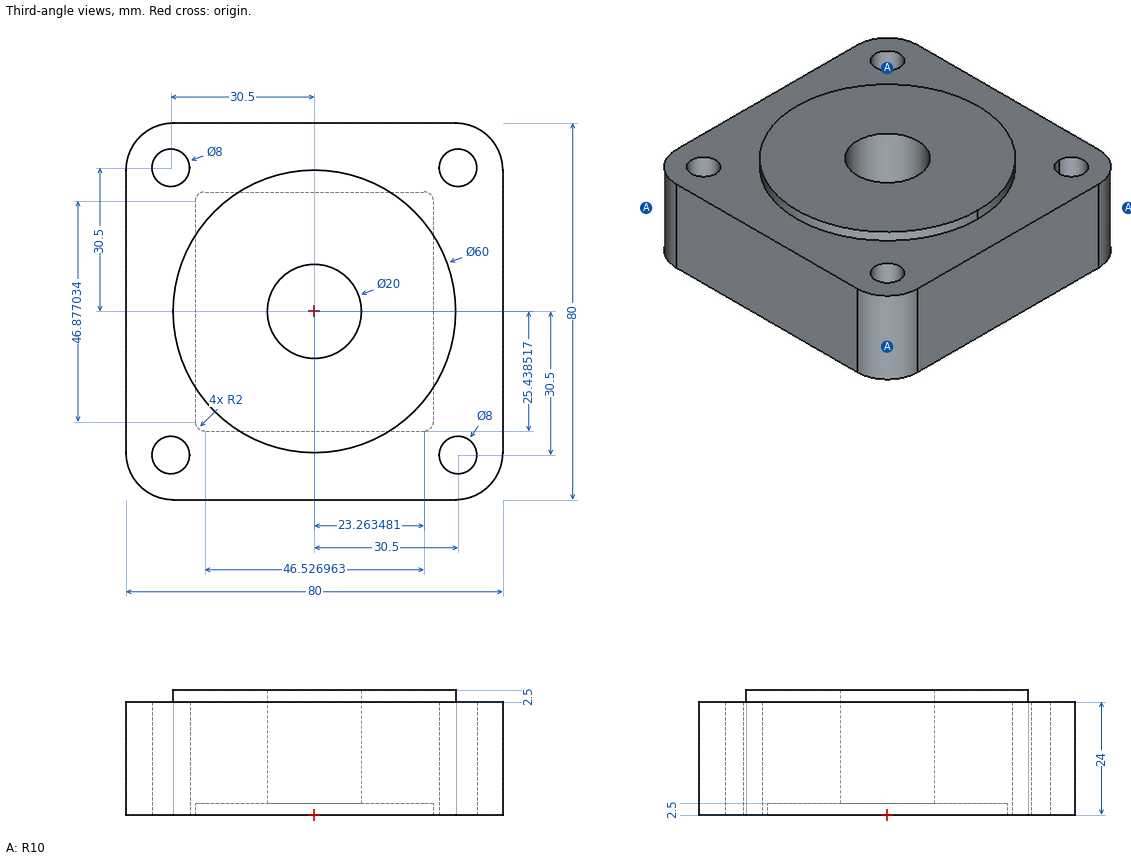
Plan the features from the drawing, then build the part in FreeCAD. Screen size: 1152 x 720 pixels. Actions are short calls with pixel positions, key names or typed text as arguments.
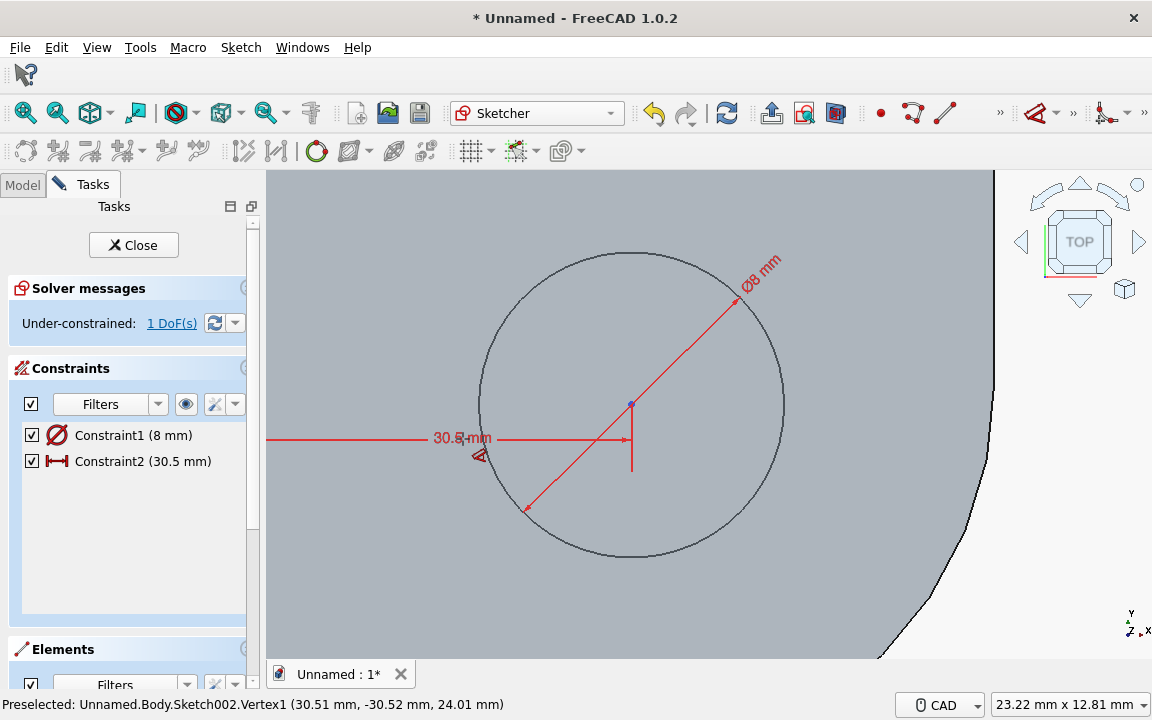
click(632, 405)
click(666, 301)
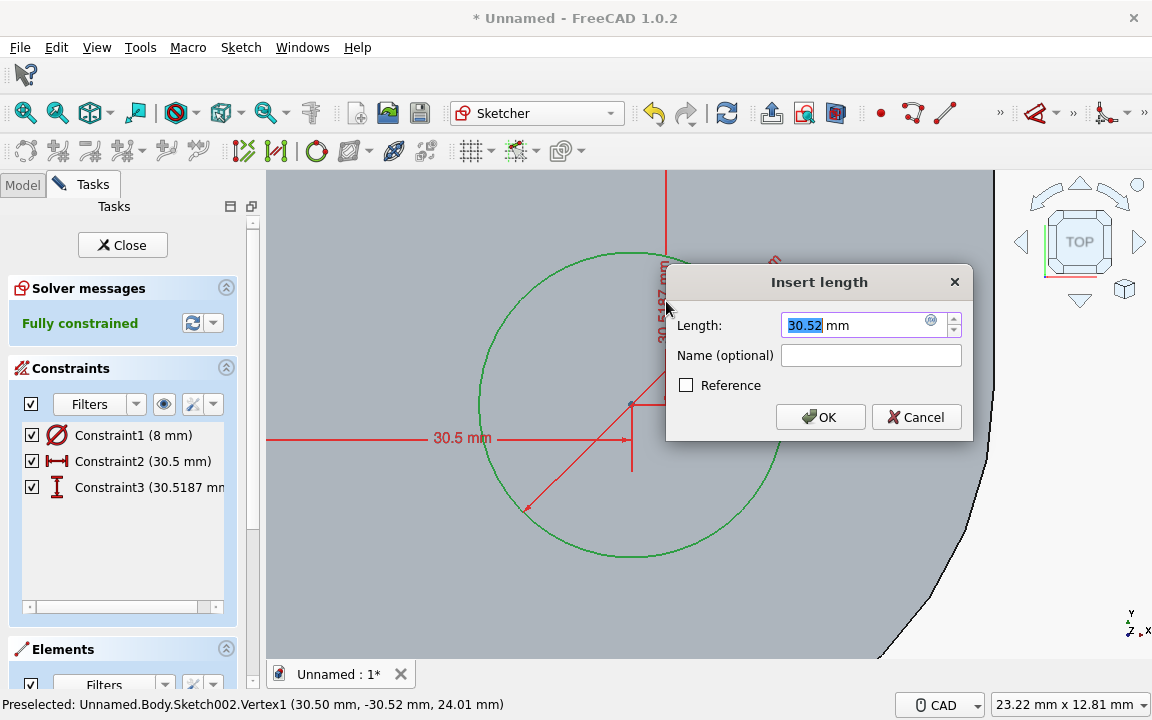
text(30.5)
key(Return)
key(Escape)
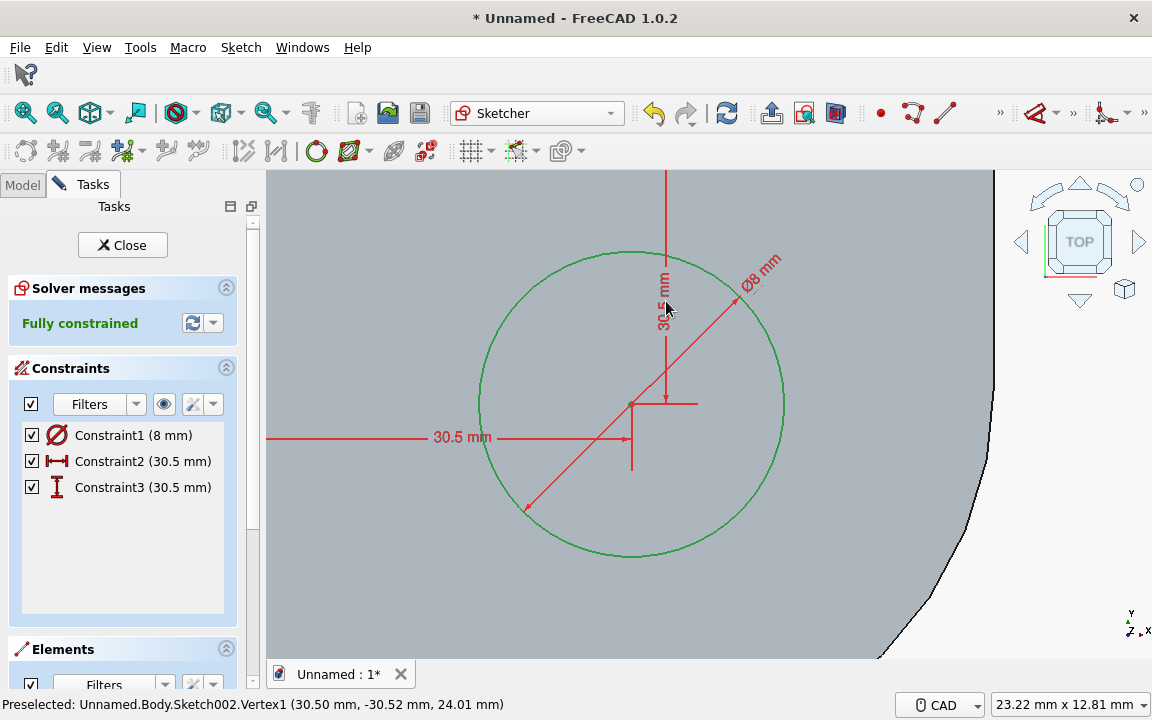
click(123, 245)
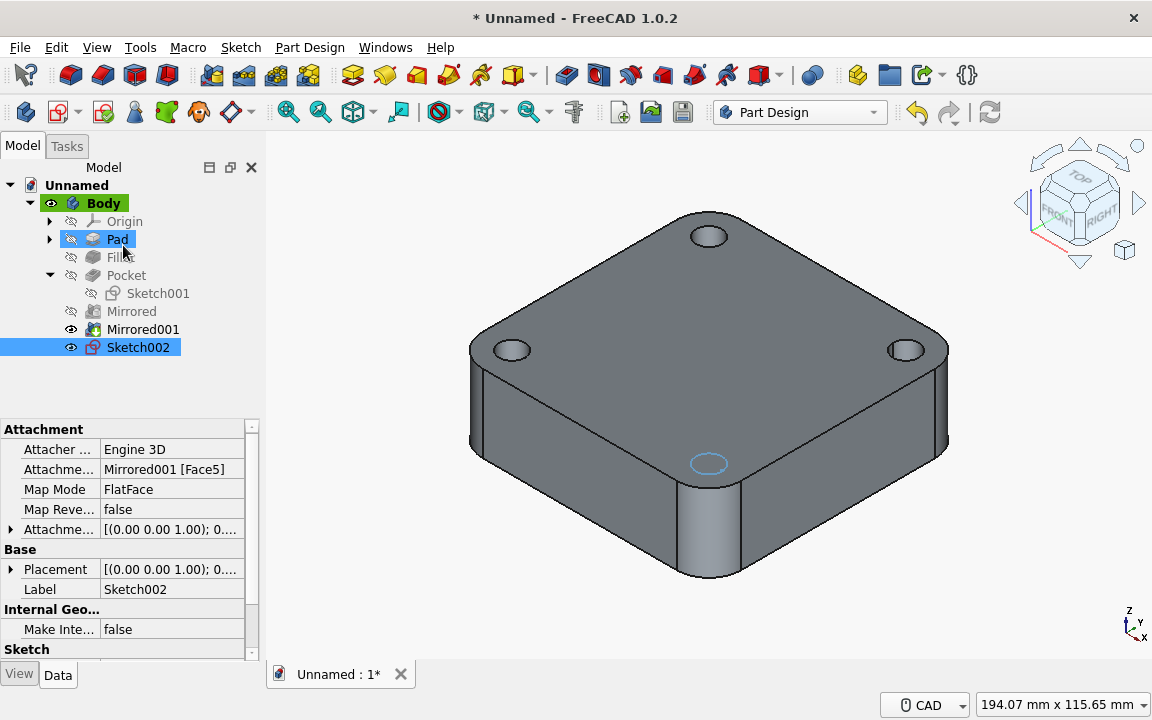
click(568, 76)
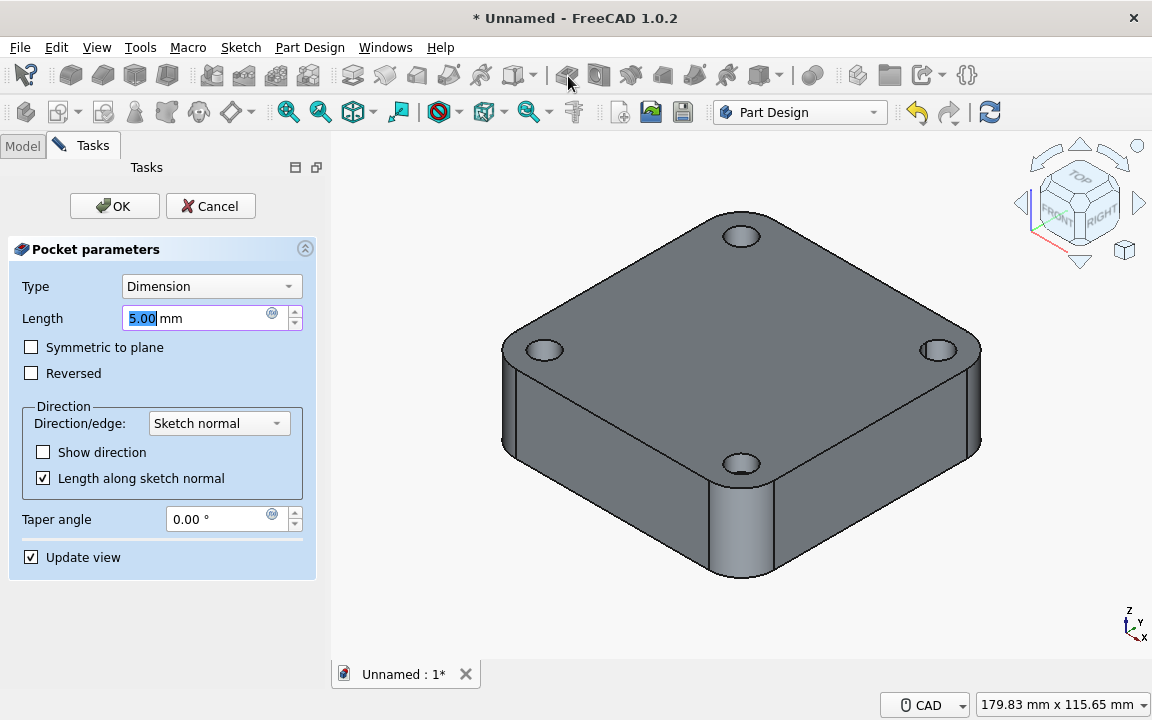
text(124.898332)
key(Tab)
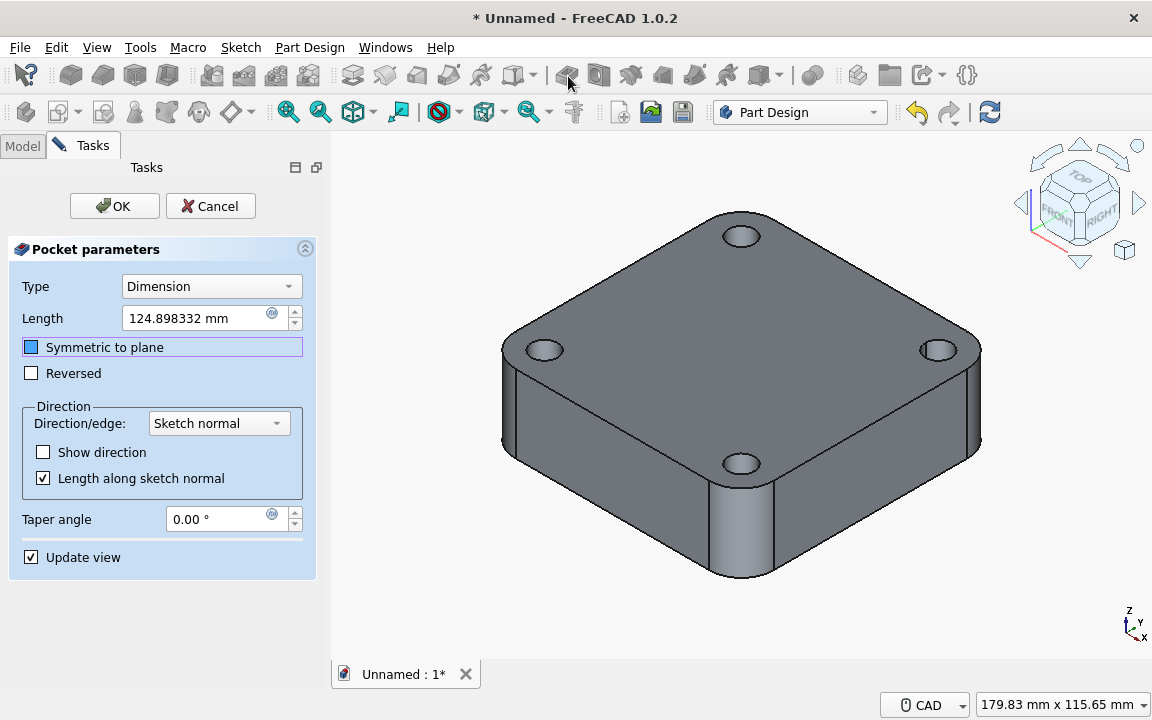
click(30, 347)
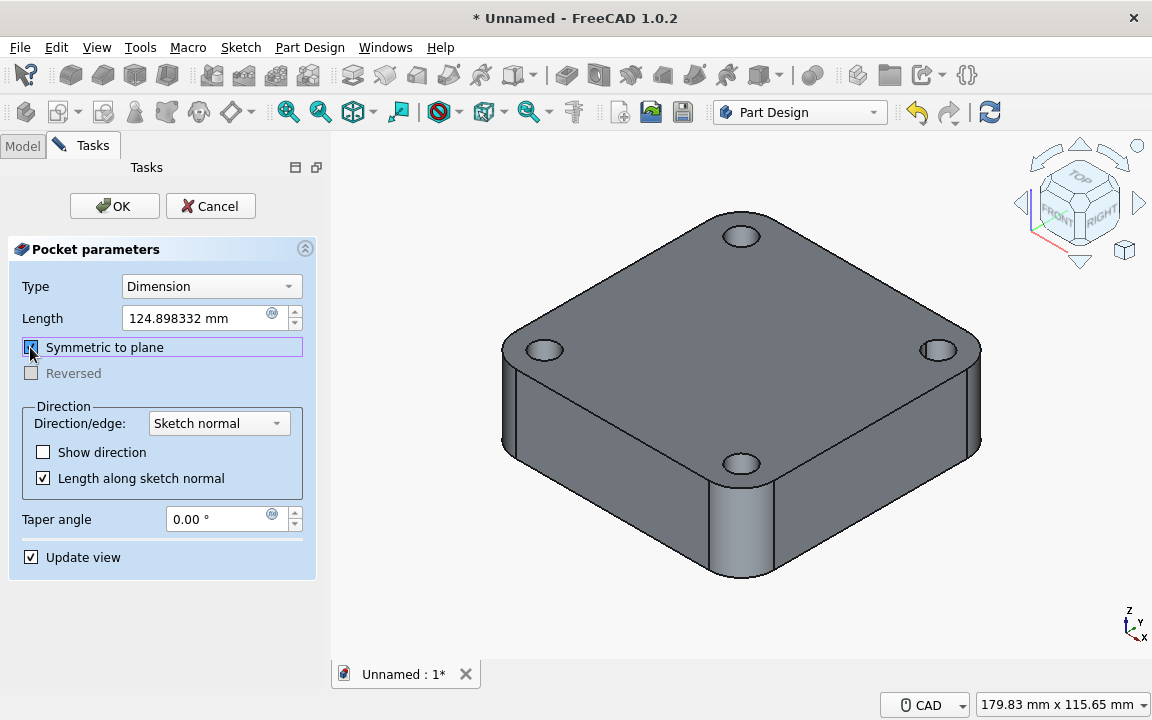
click(115, 206)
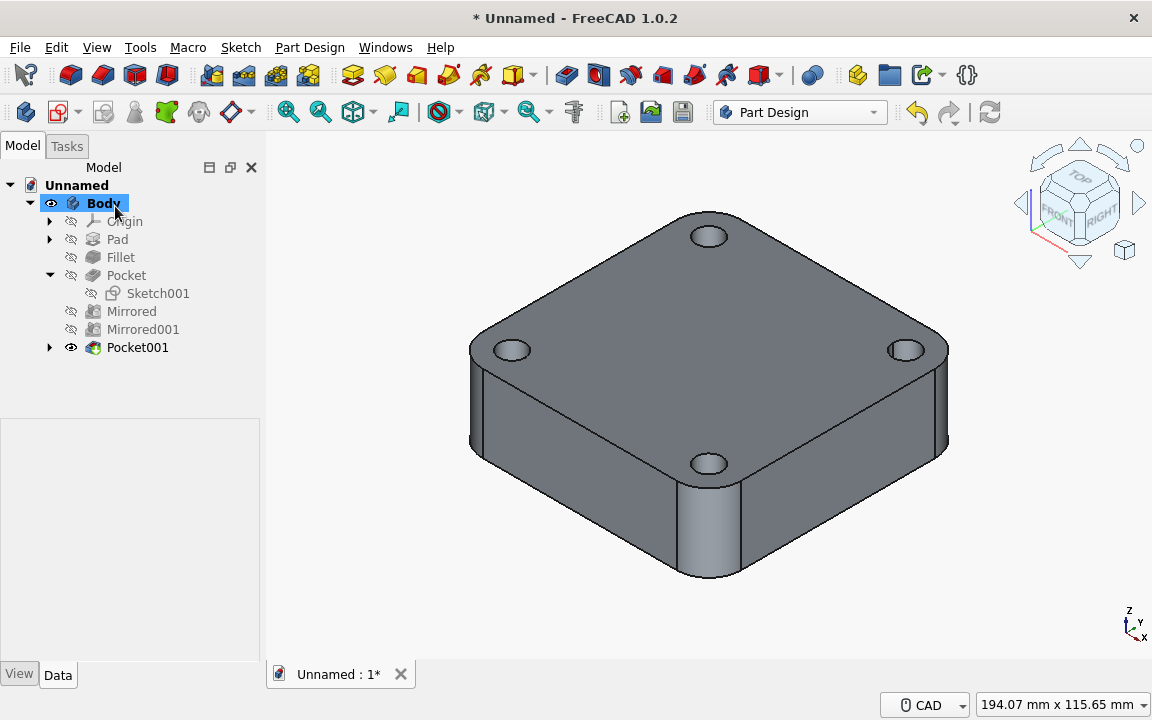
click(709, 349)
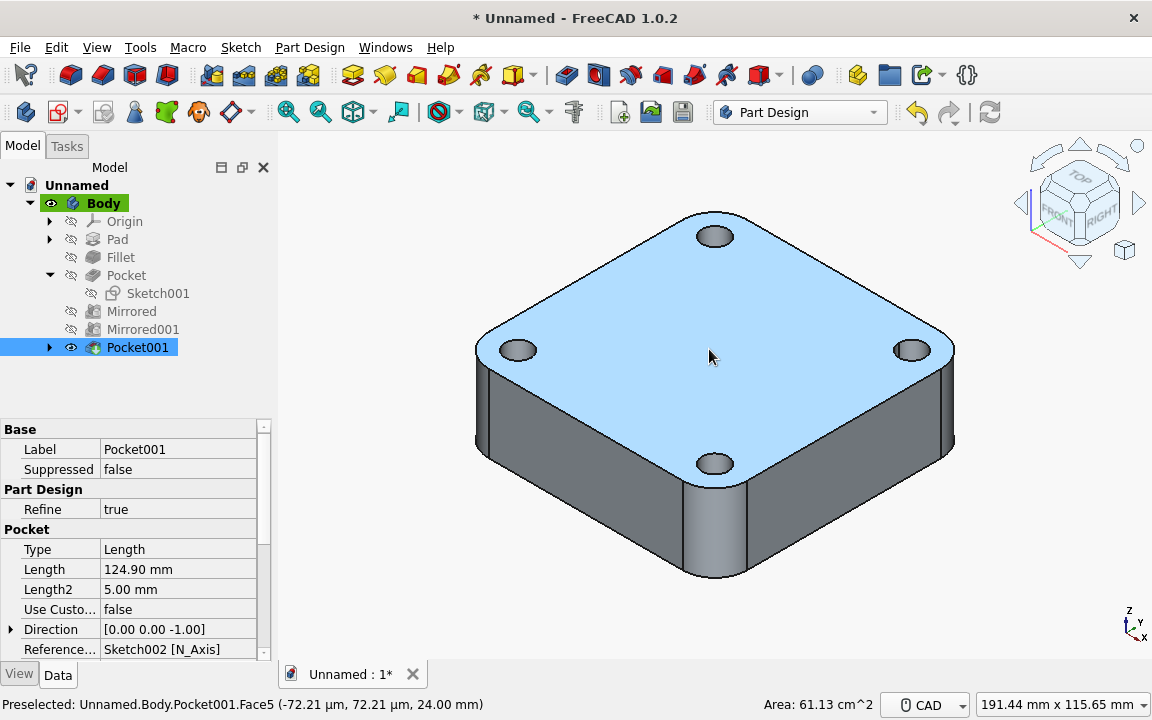
click(58, 112)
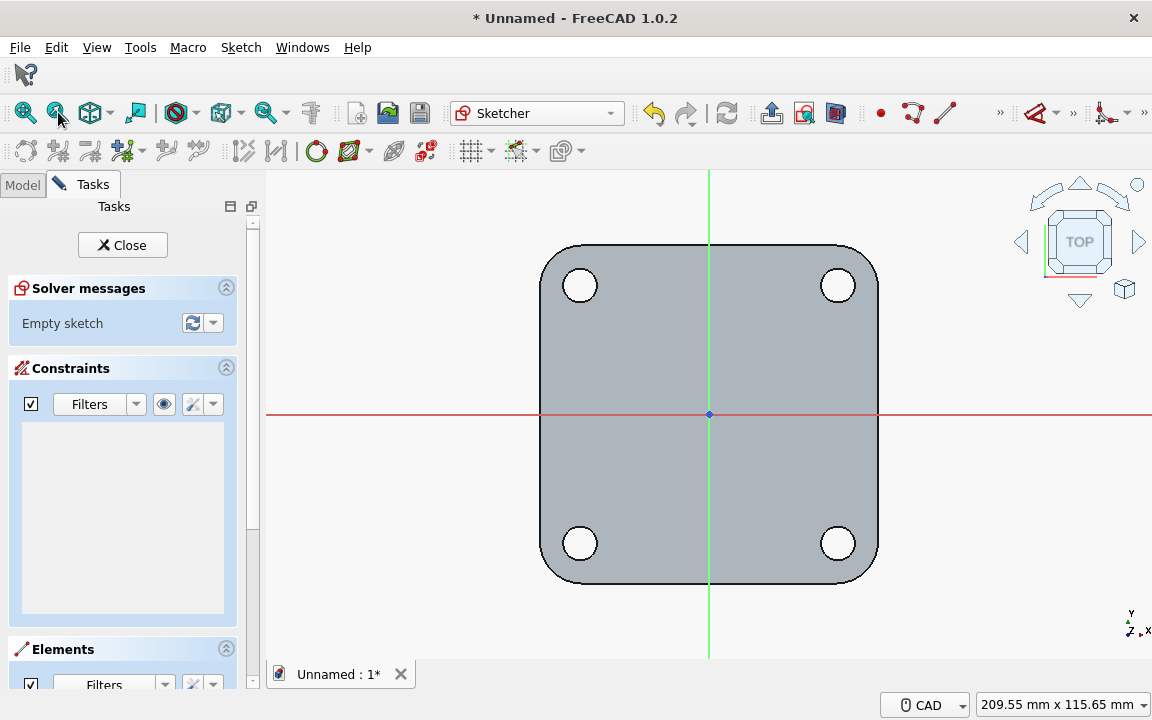
key(g)
key(c)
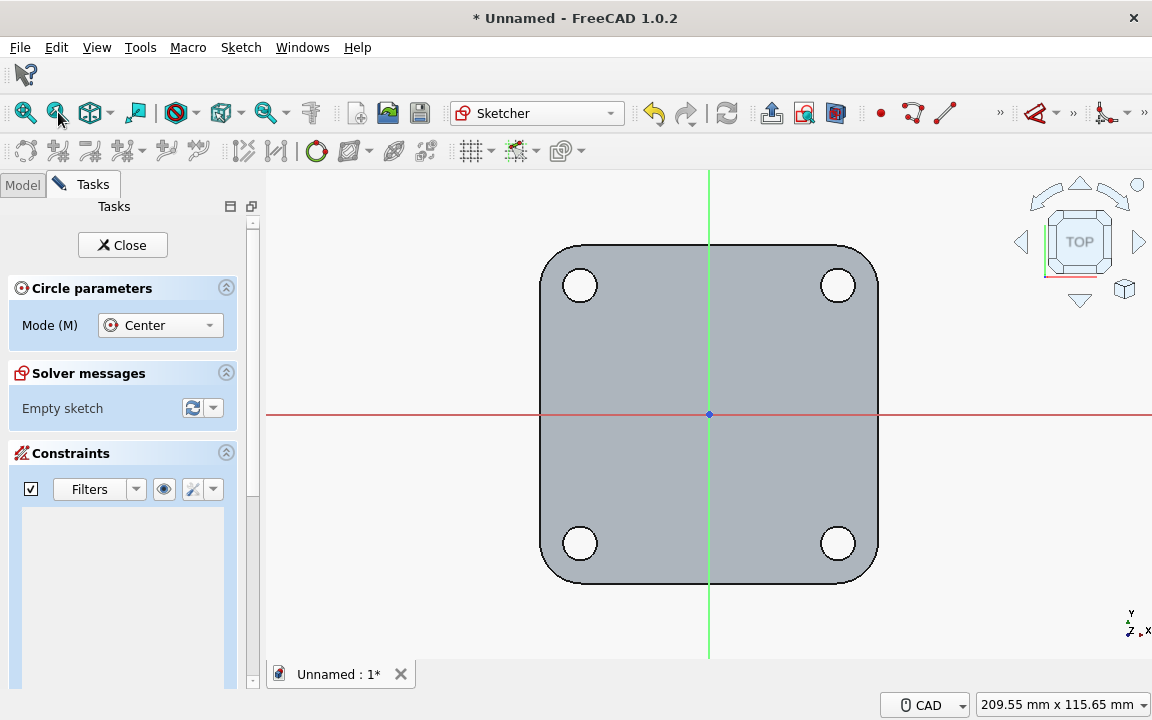
click(709, 414)
click(799, 325)
key(Escape)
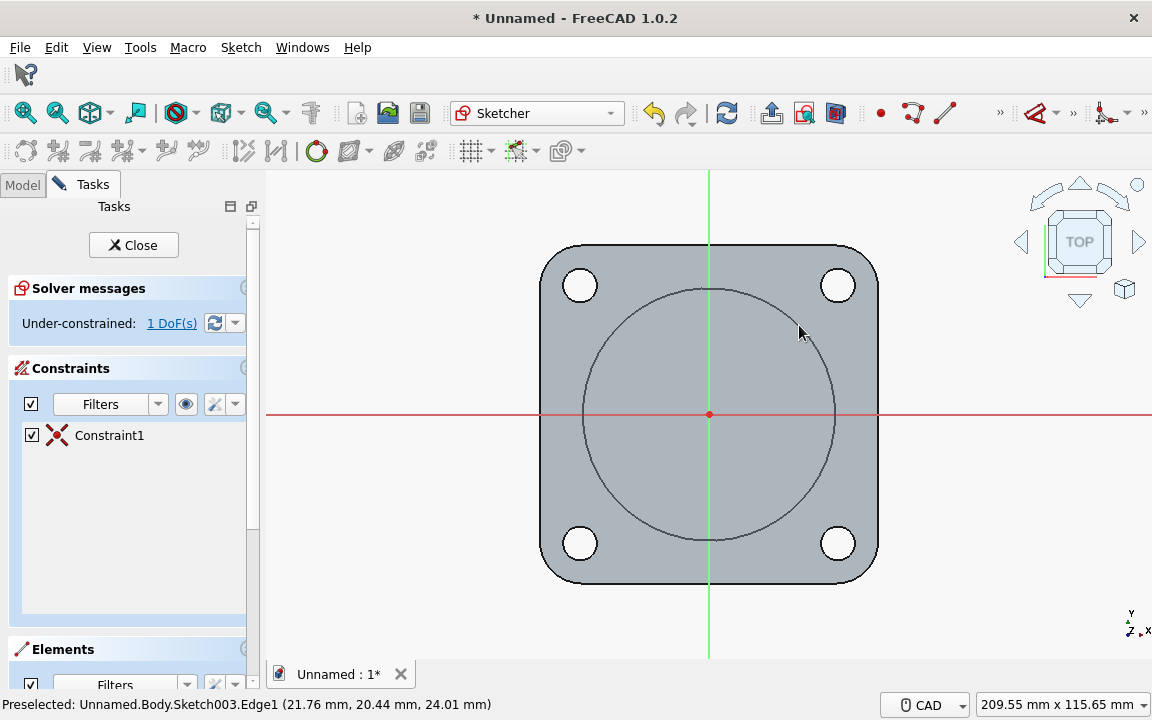
click(1036, 114)